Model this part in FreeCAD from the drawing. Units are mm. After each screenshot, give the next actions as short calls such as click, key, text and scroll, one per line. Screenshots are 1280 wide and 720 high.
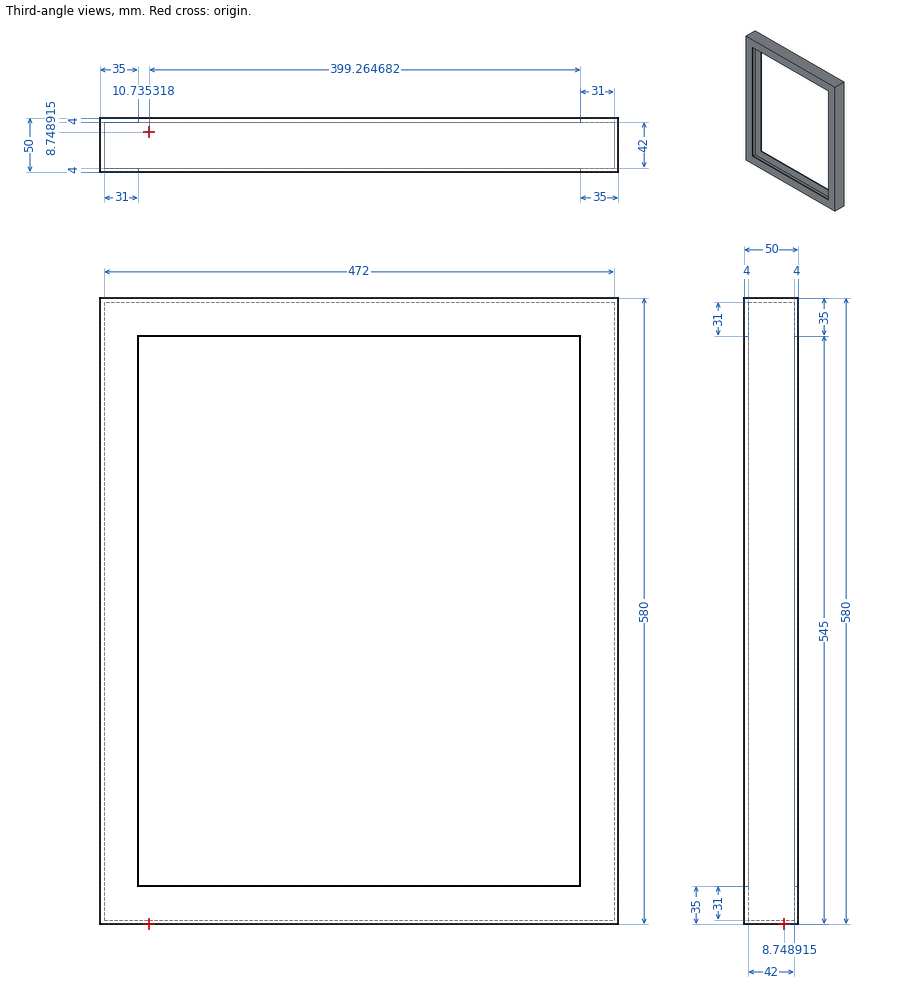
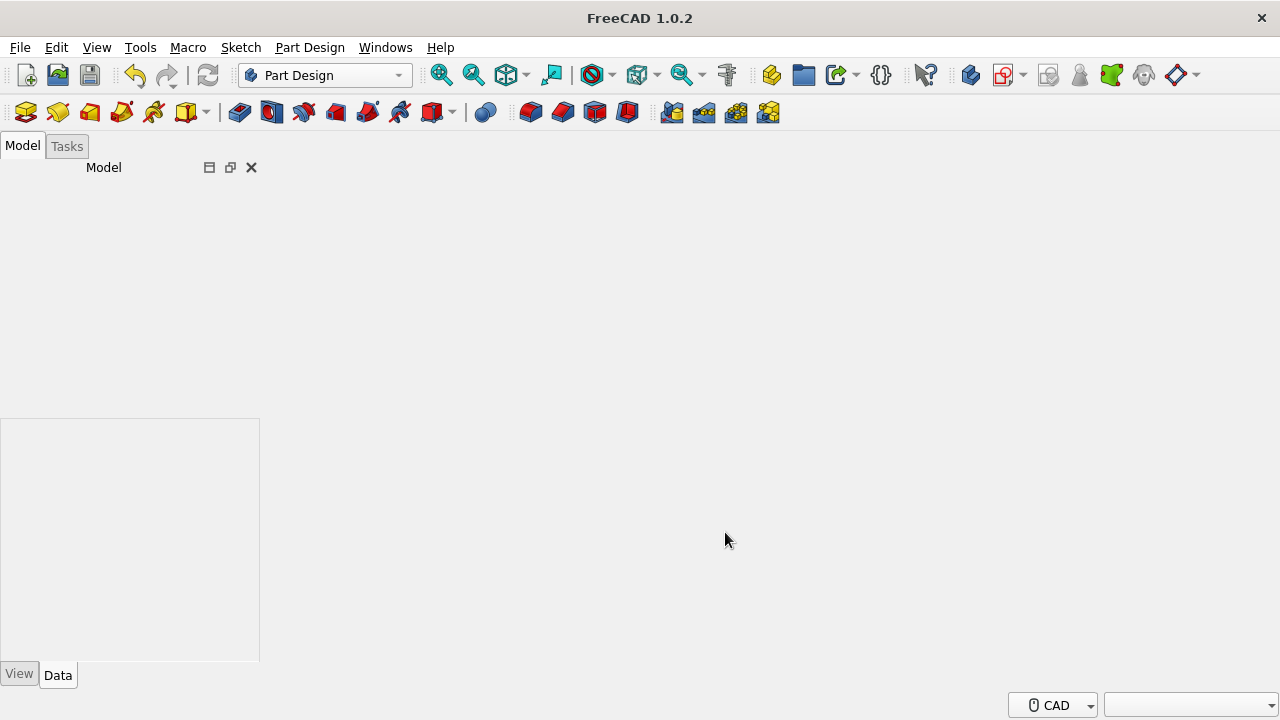
click(26, 76)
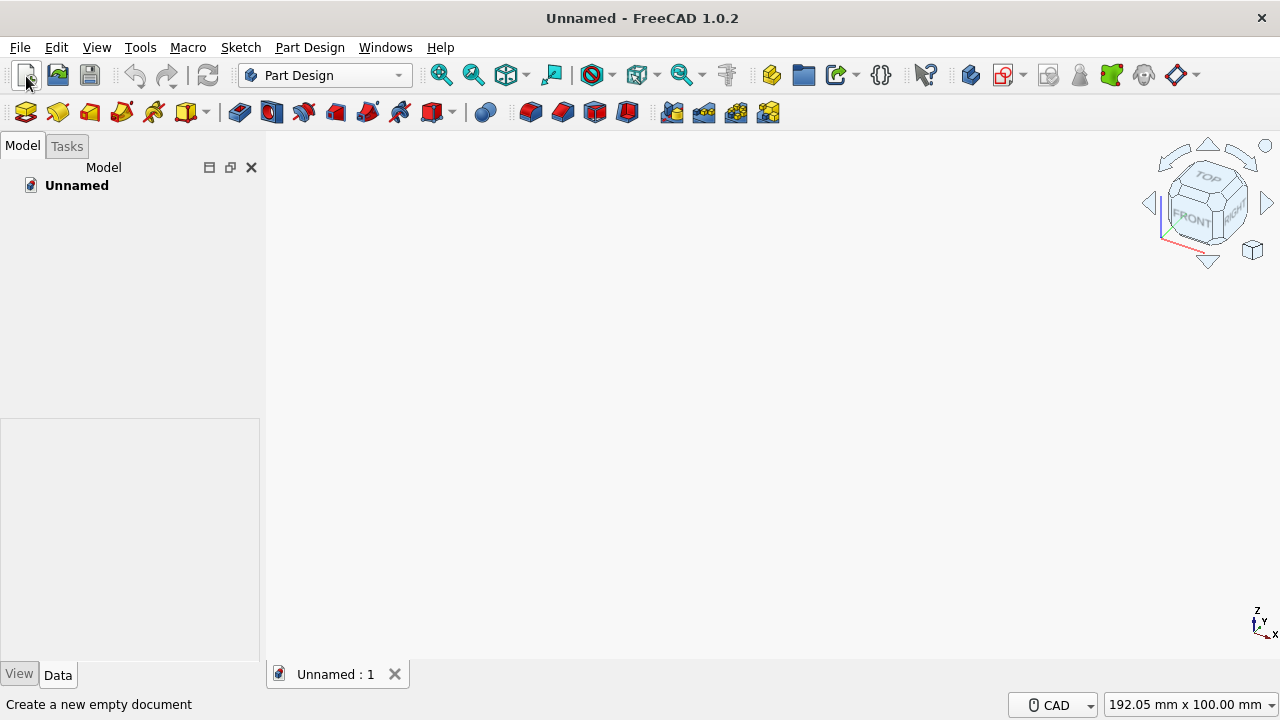
click(1004, 76)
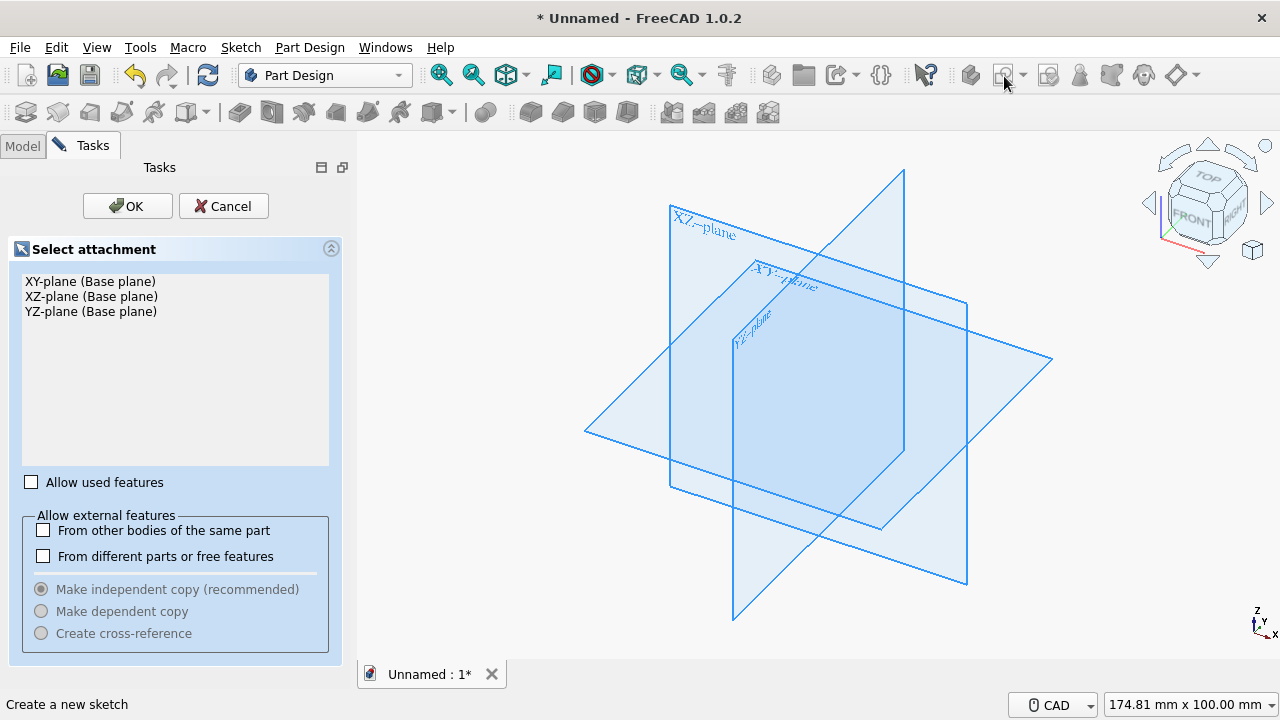
click(82, 282)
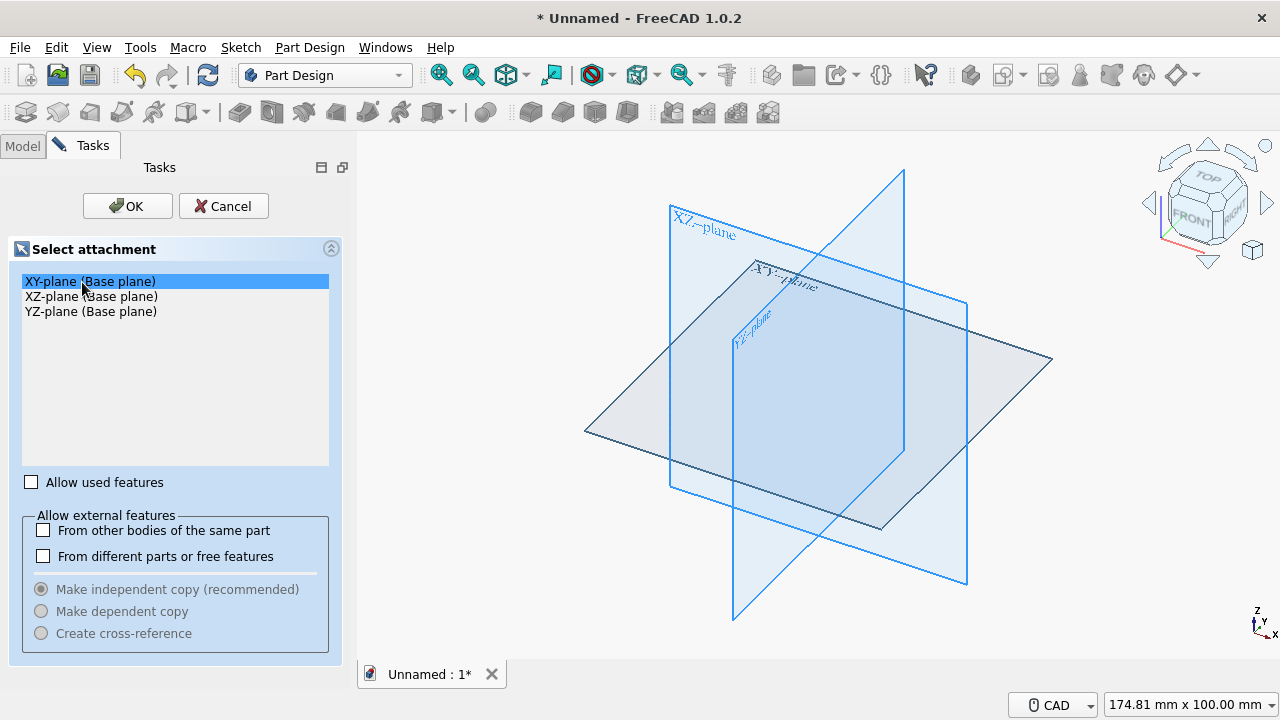
click(128, 206)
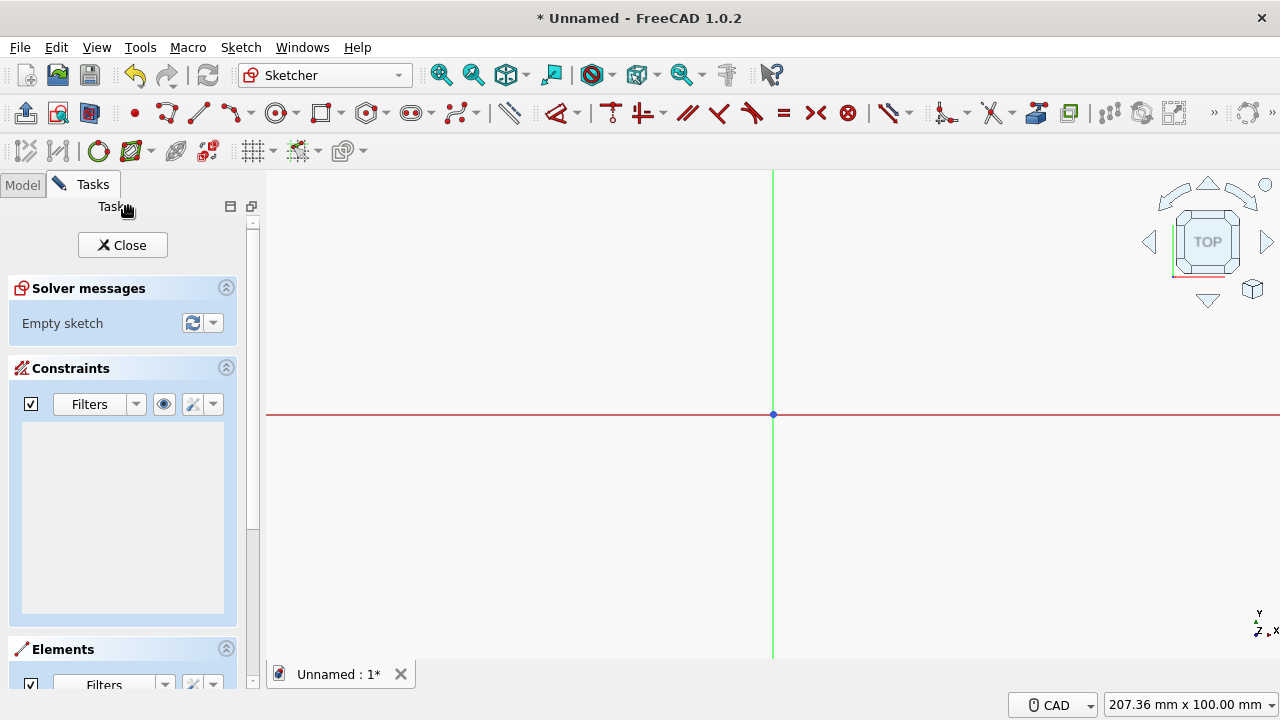
key(g)
key(m)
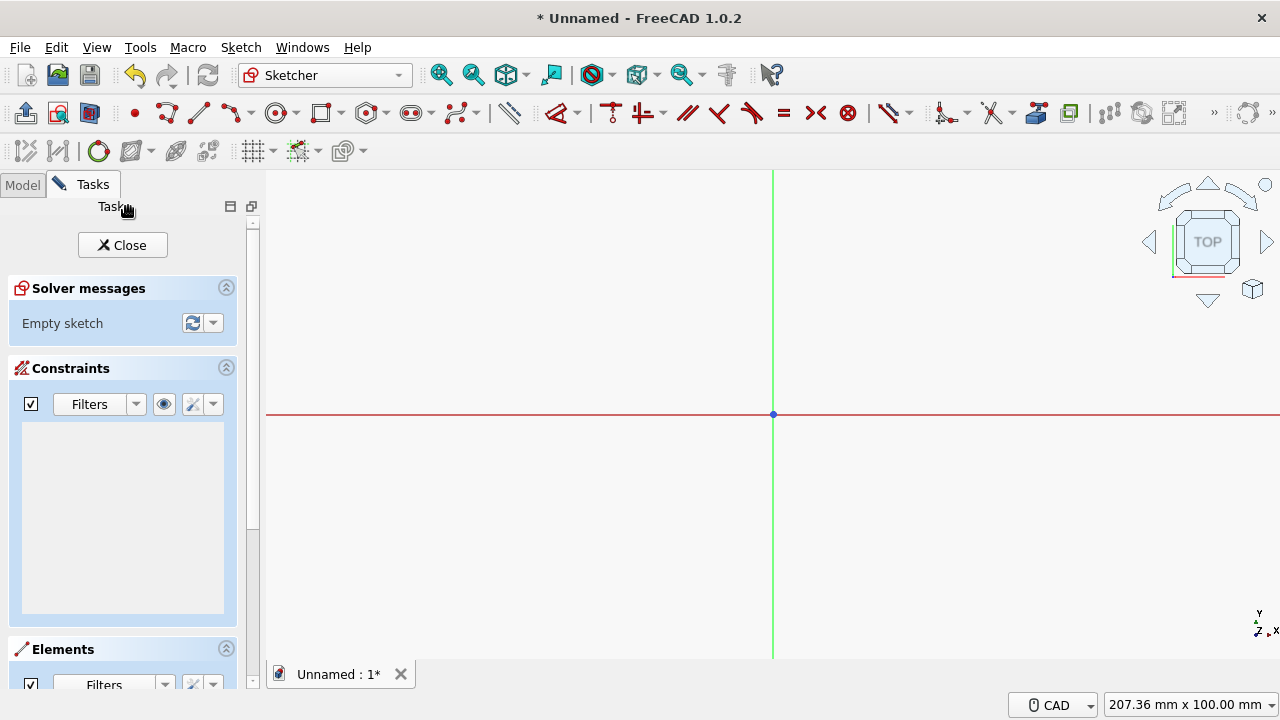
click(721, 372)
click(721, 352)
click(549, 352)
click(549, 597)
click(721, 597)
click(721, 577)
click(569, 577)
click(569, 372)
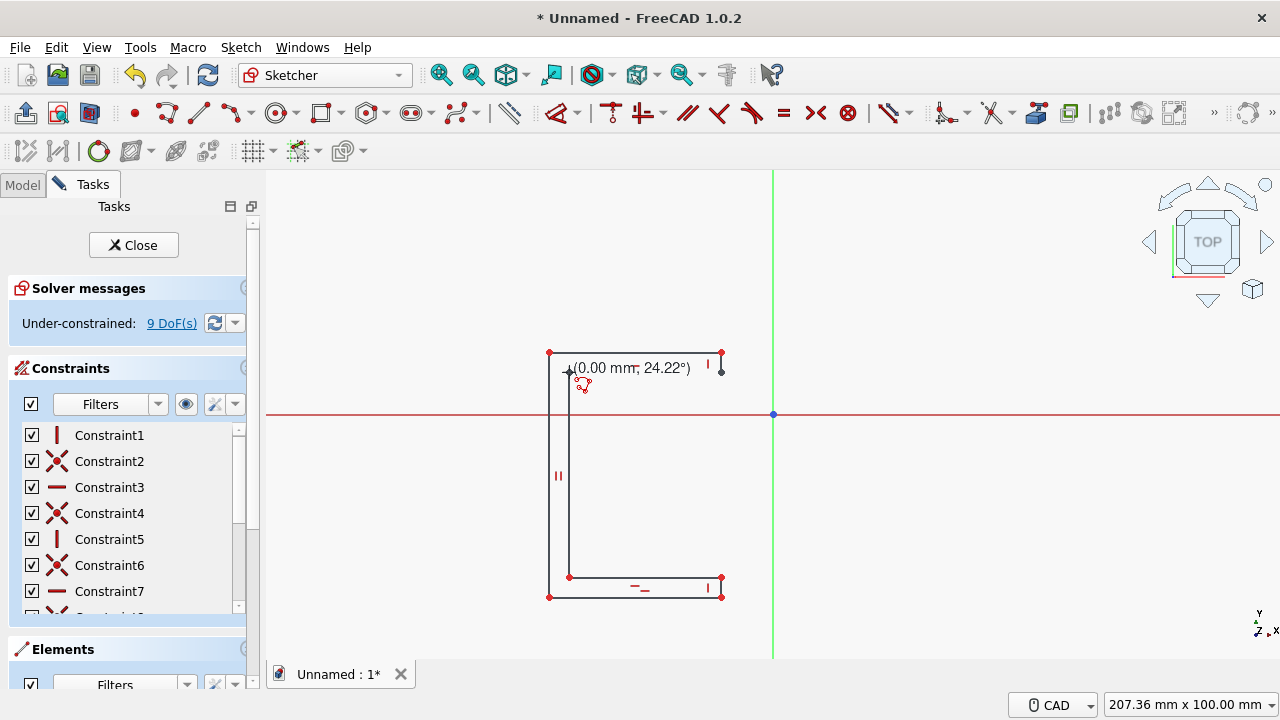
scroll(721, 372, up, 3)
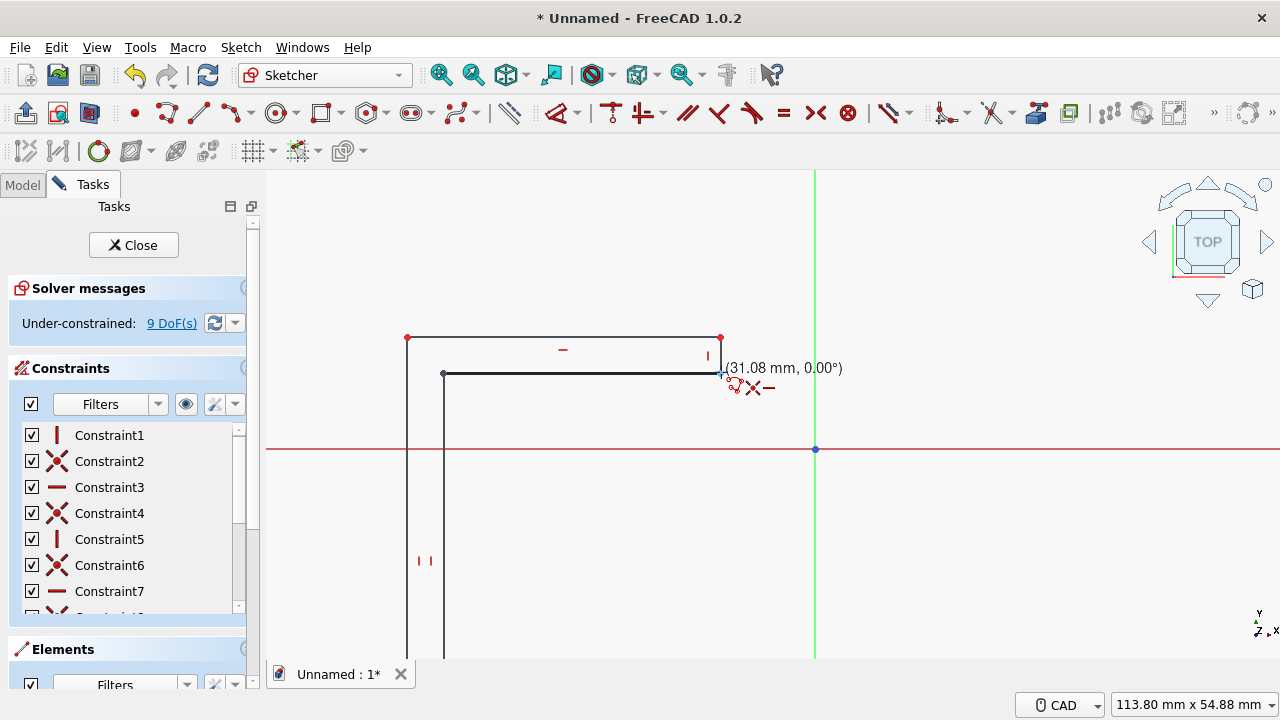
click(721, 373)
key(Escape)
key(Escape)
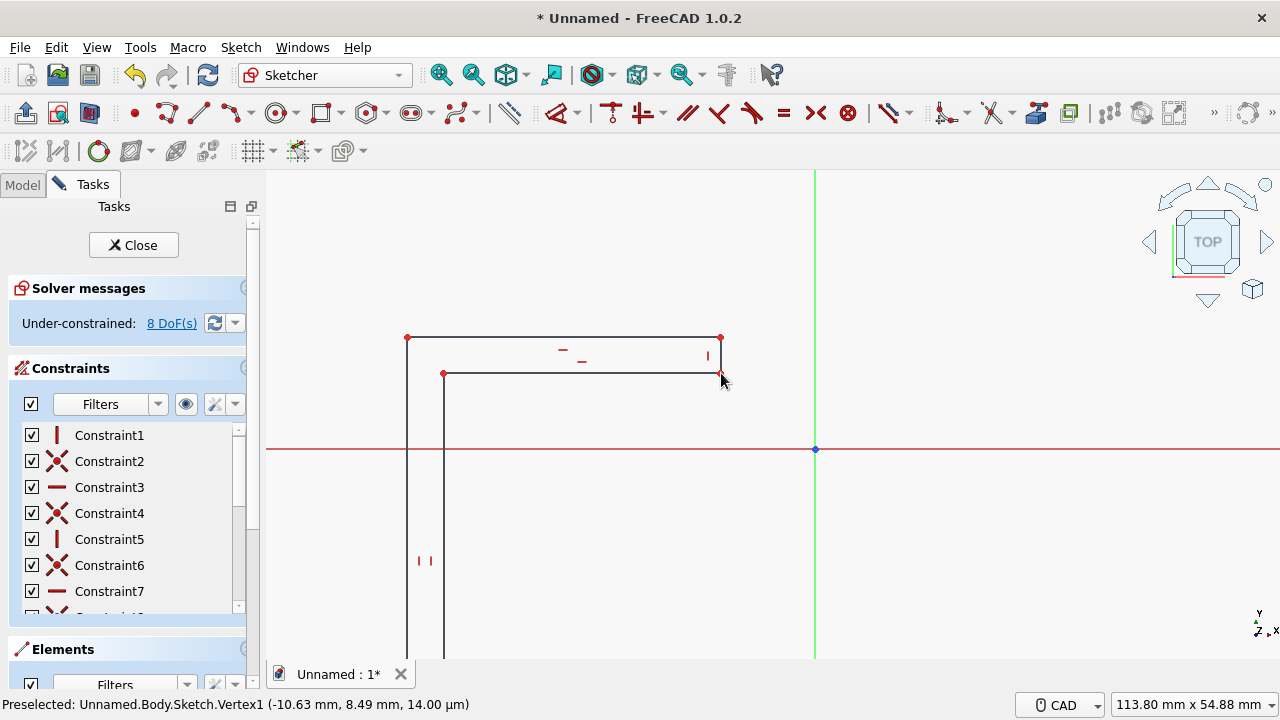
click(556, 114)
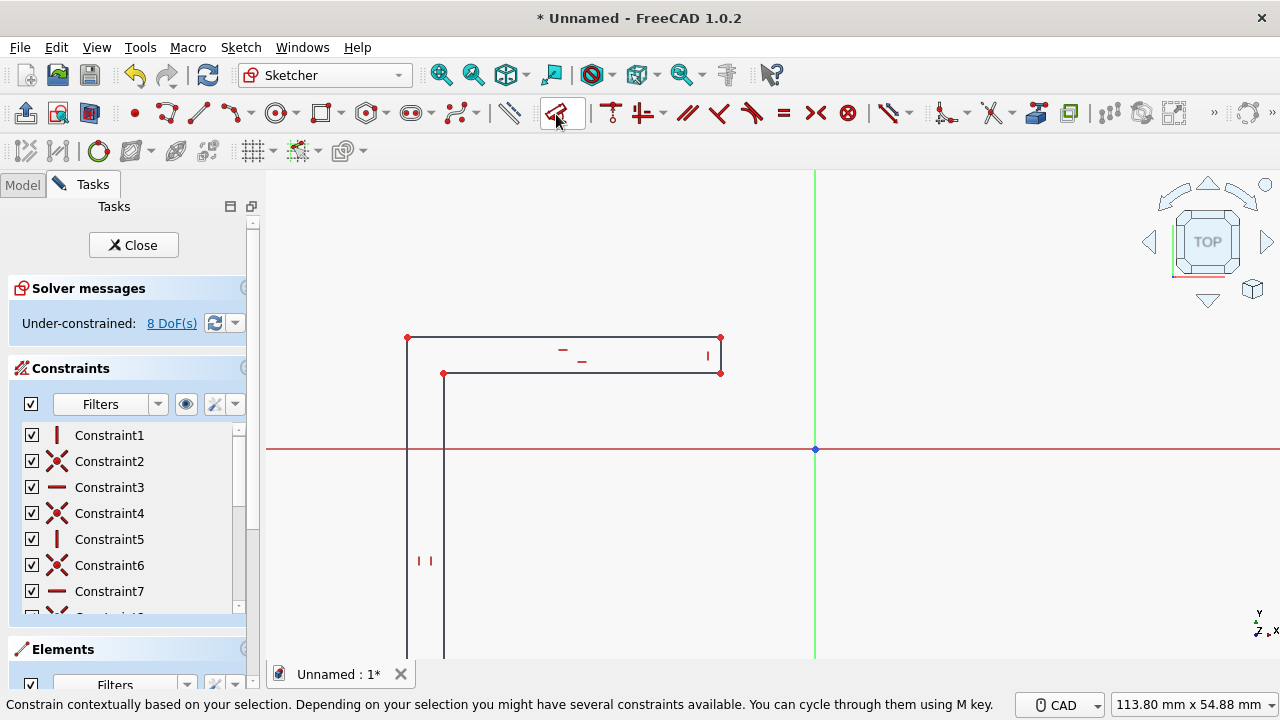
scroll(721, 363, up, 2)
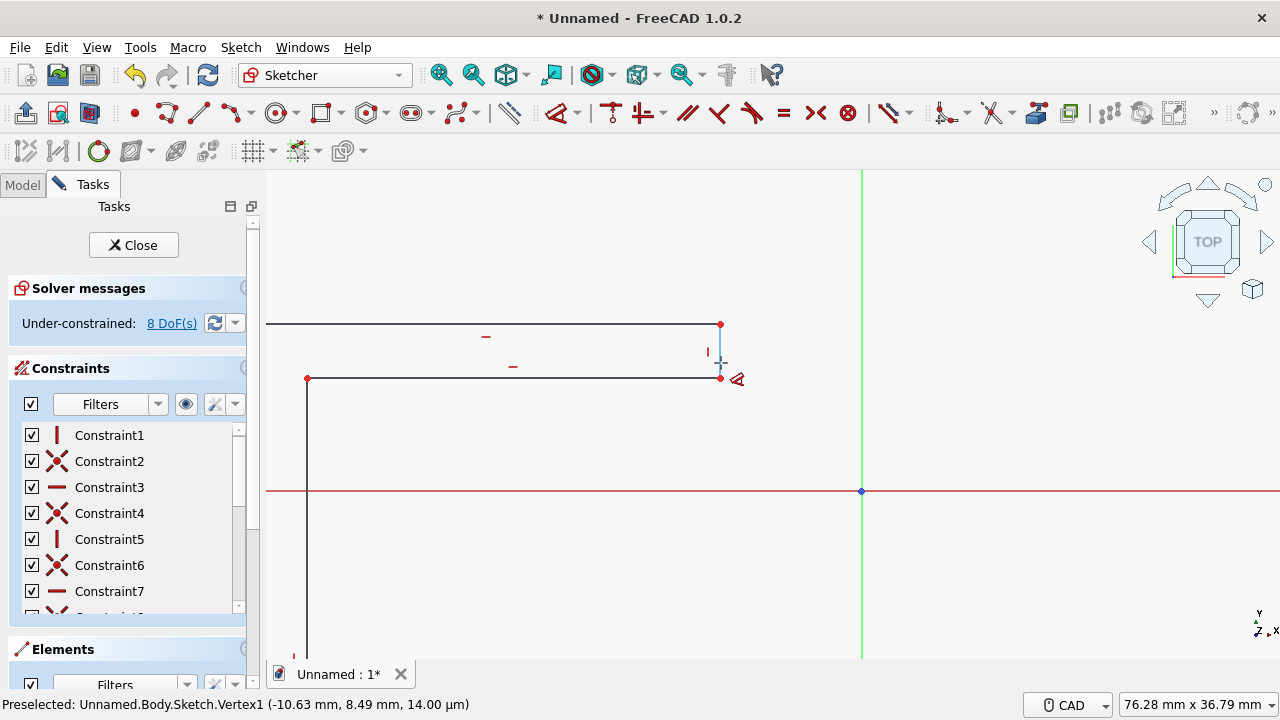
click(720, 362)
click(754, 351)